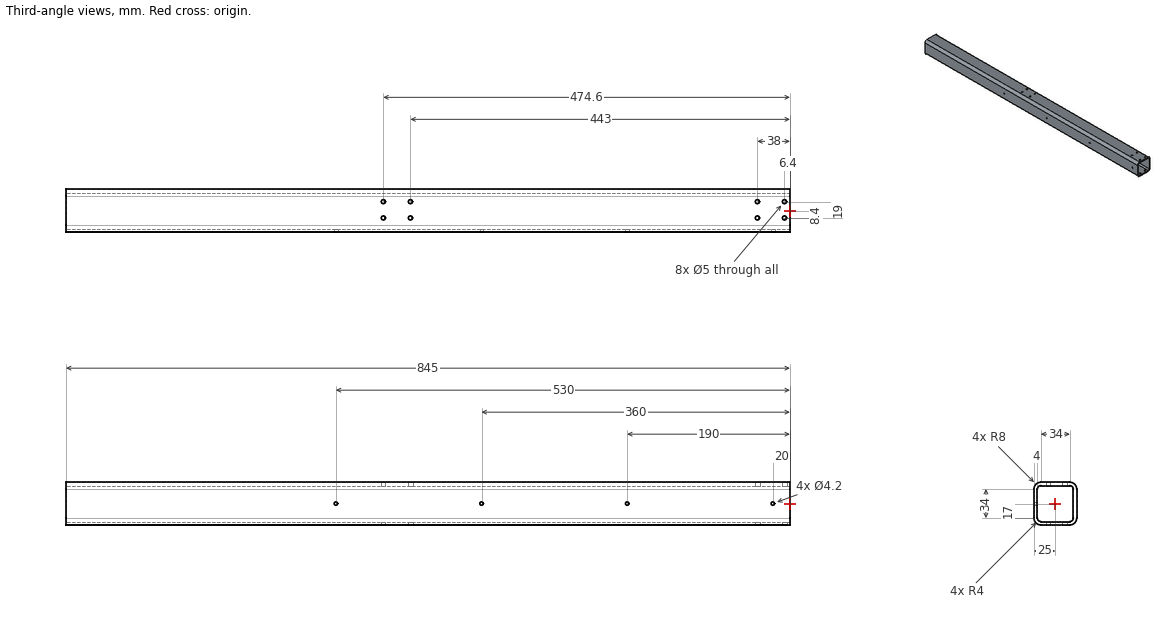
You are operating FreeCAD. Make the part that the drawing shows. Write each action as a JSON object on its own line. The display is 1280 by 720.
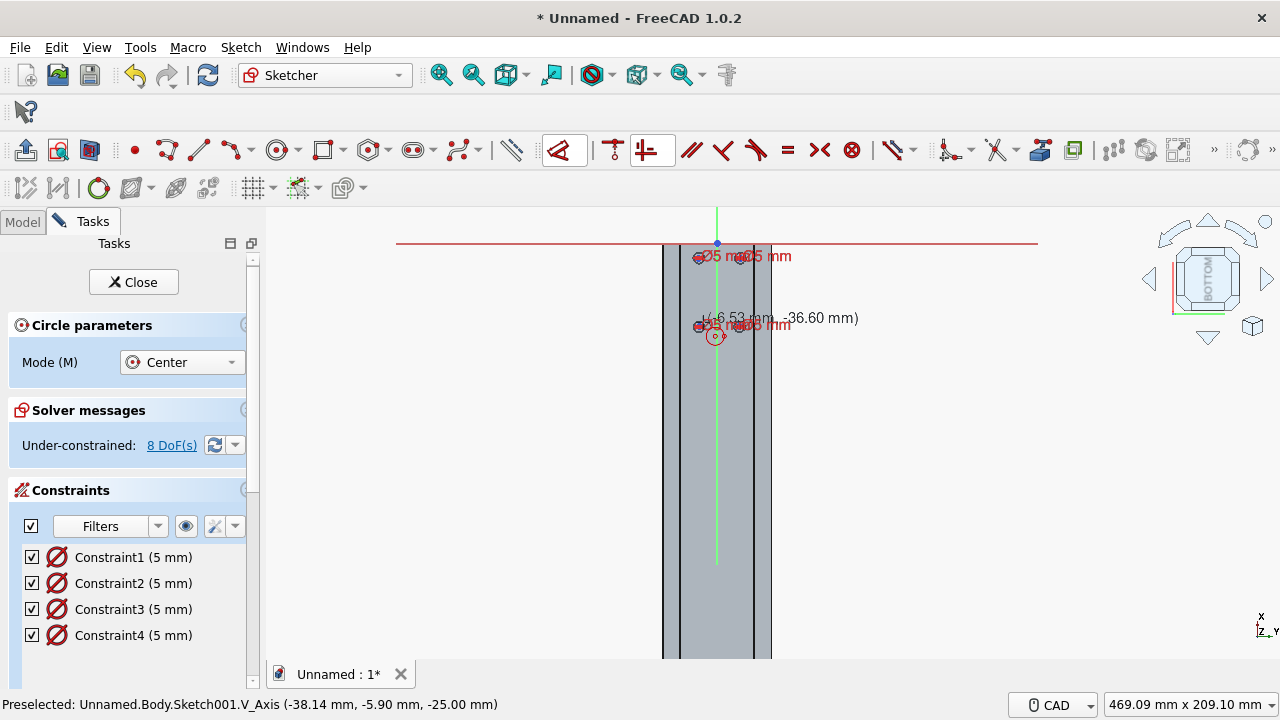
{"action": "scroll", "coordinate": [700, 326], "scroll_direction": "down", "scroll_amount": 7}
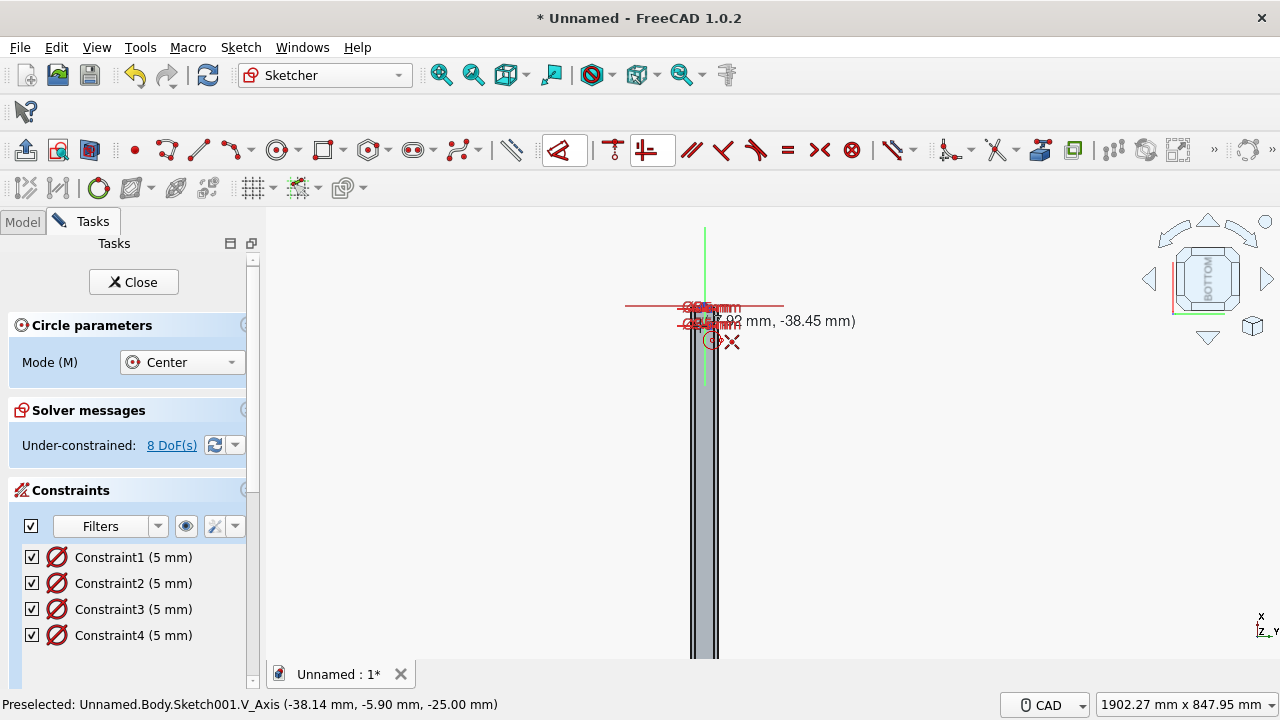
{"action": "scroll", "coordinate": [710, 542], "scroll_direction": "up", "scroll_amount": 15}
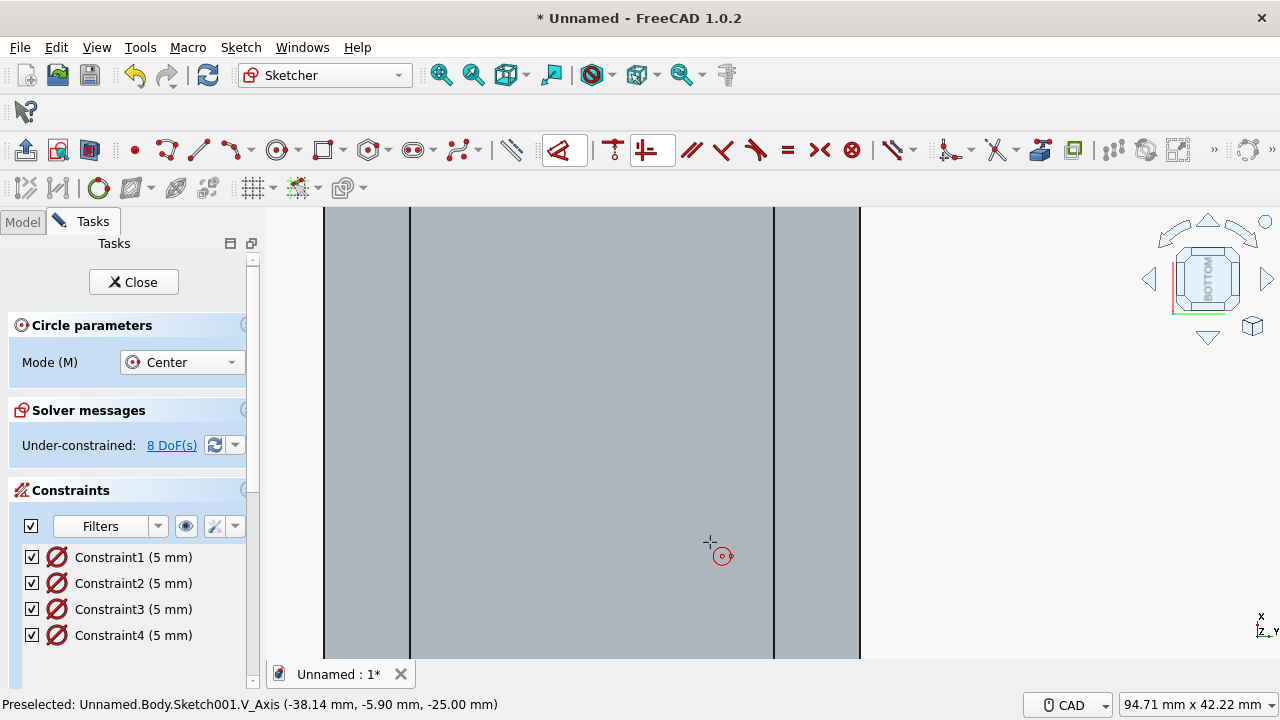
{"action": "scroll", "coordinate": [710, 543], "scroll_direction": "down", "scroll_amount": 15}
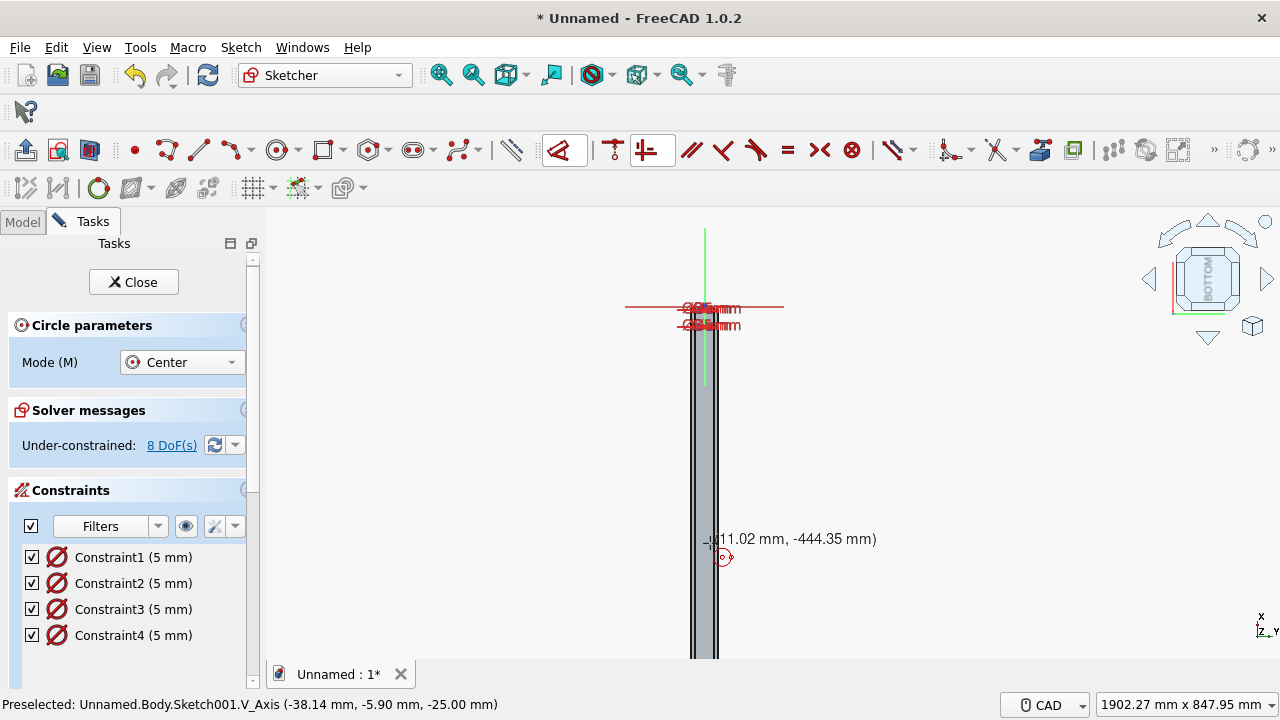
{"action": "scroll", "coordinate": [710, 543], "scroll_direction": "up", "scroll_amount": 6}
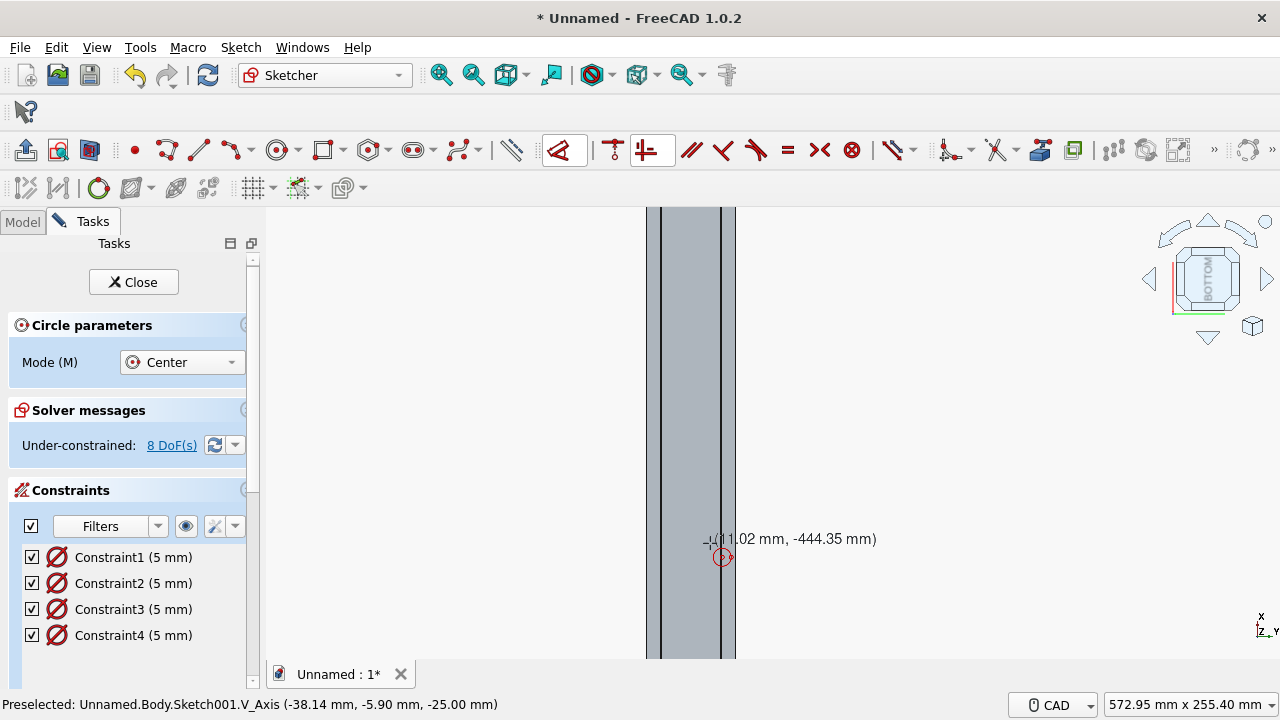
{"action": "left_click", "coordinate": [710, 541]}
{"action": "mouse_move", "coordinate": [713, 538]}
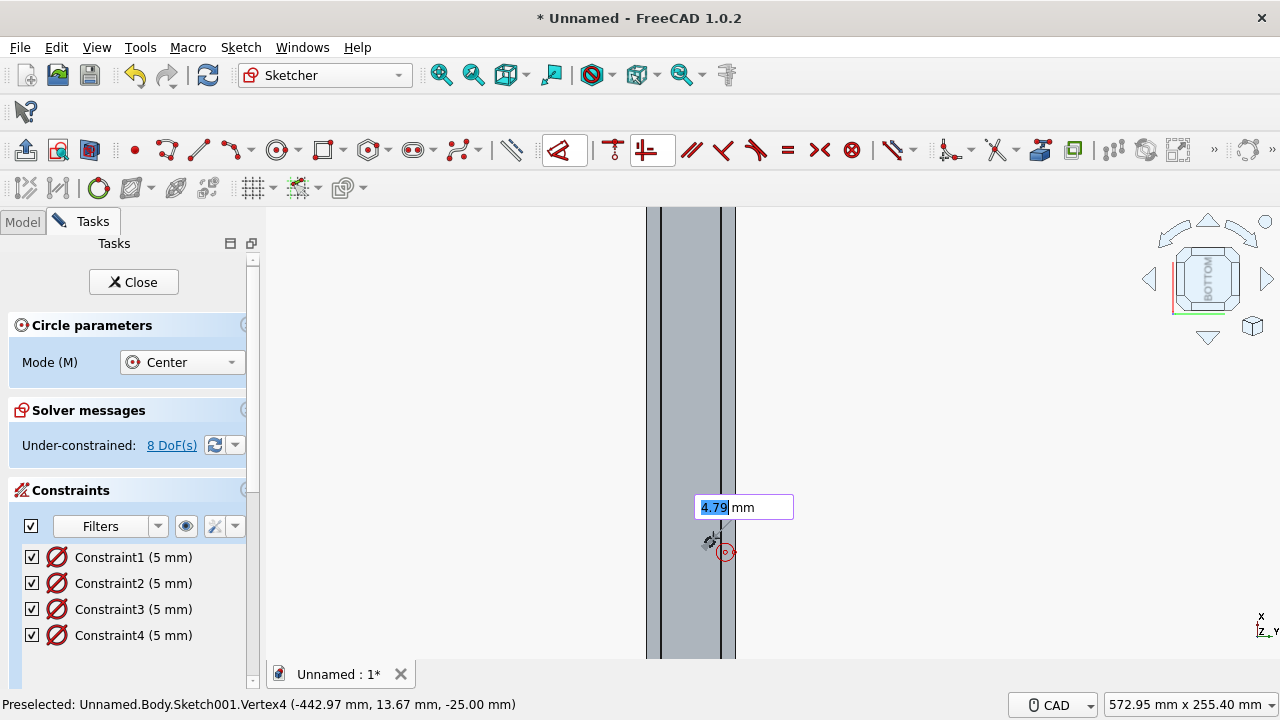
{"action": "type", "text": "5"}
{"action": "key", "text": "Return"}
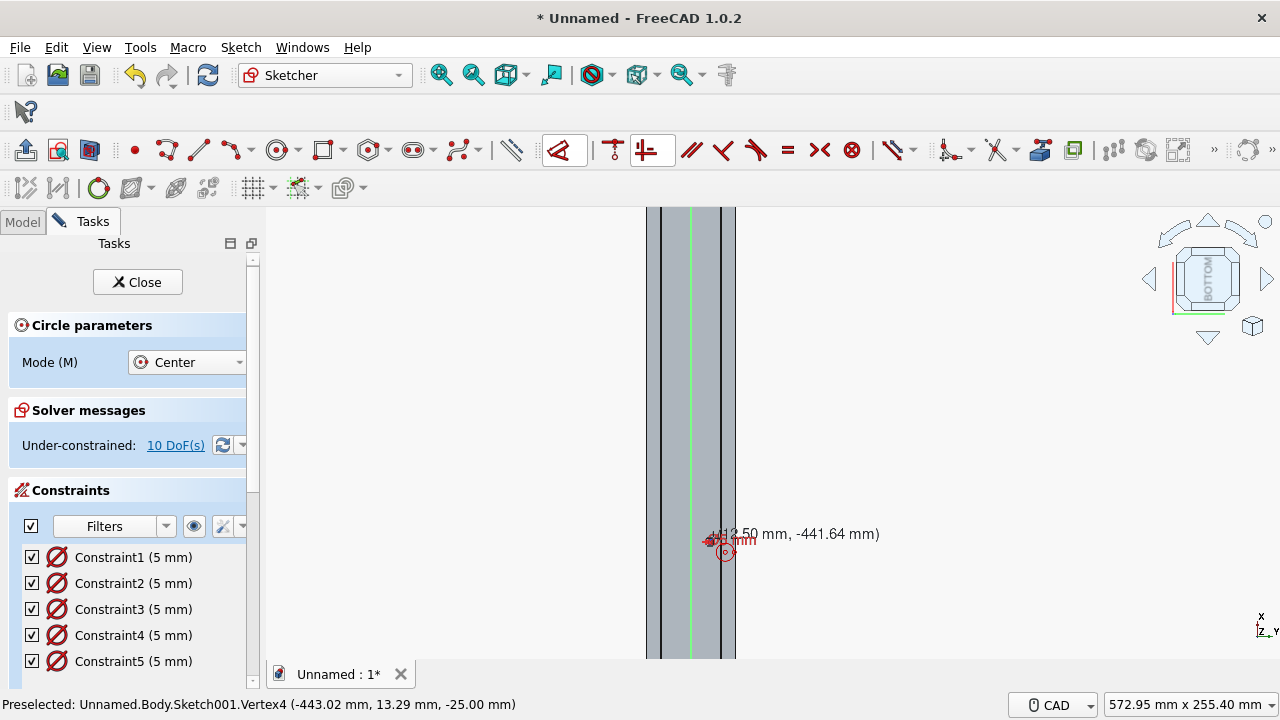
{"action": "scroll", "coordinate": [676, 541], "scroll_direction": "up", "scroll_amount": 9}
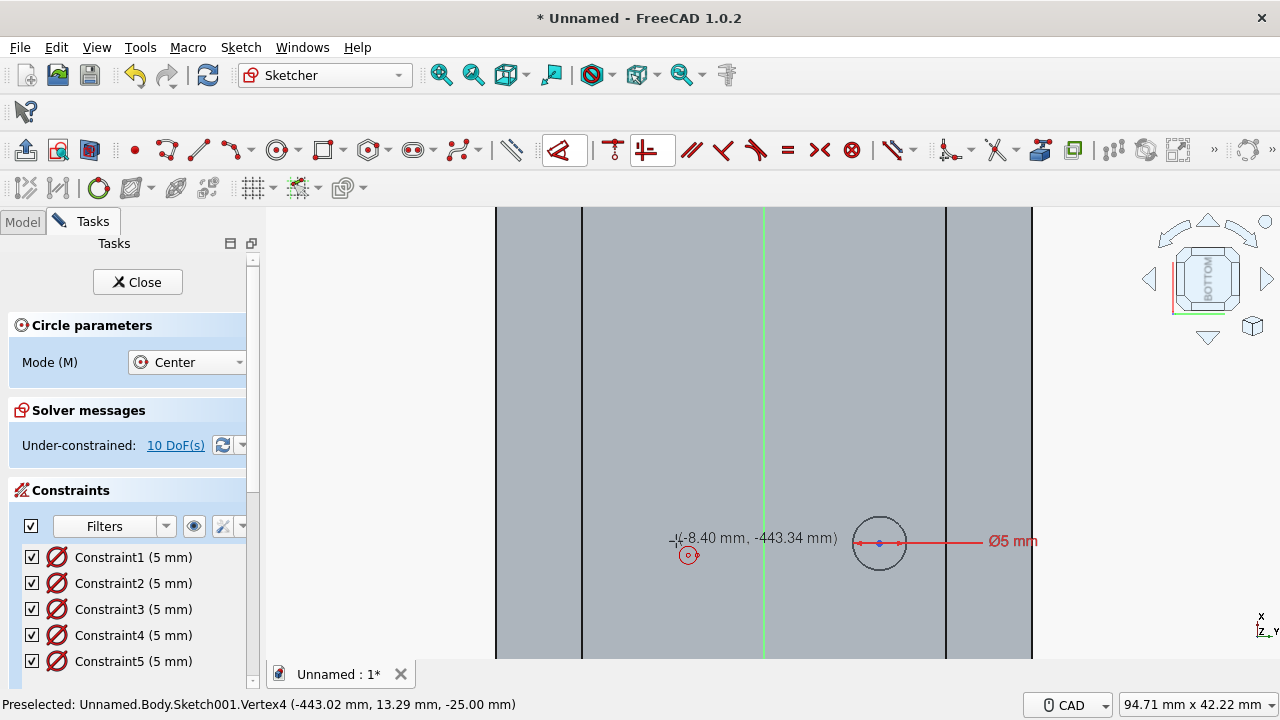
{"action": "scroll", "coordinate": [701, 542], "scroll_direction": "down", "scroll_amount": 15}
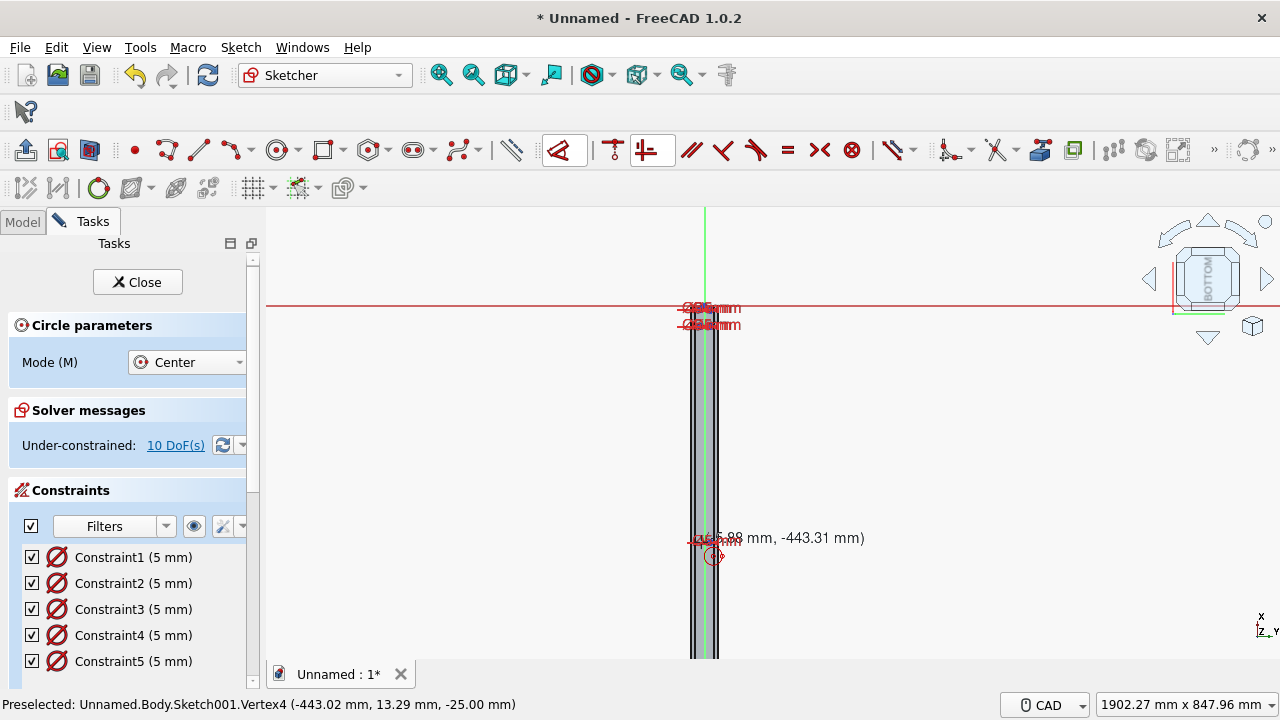
{"action": "scroll", "coordinate": [700, 543], "scroll_direction": "up", "scroll_amount": 7}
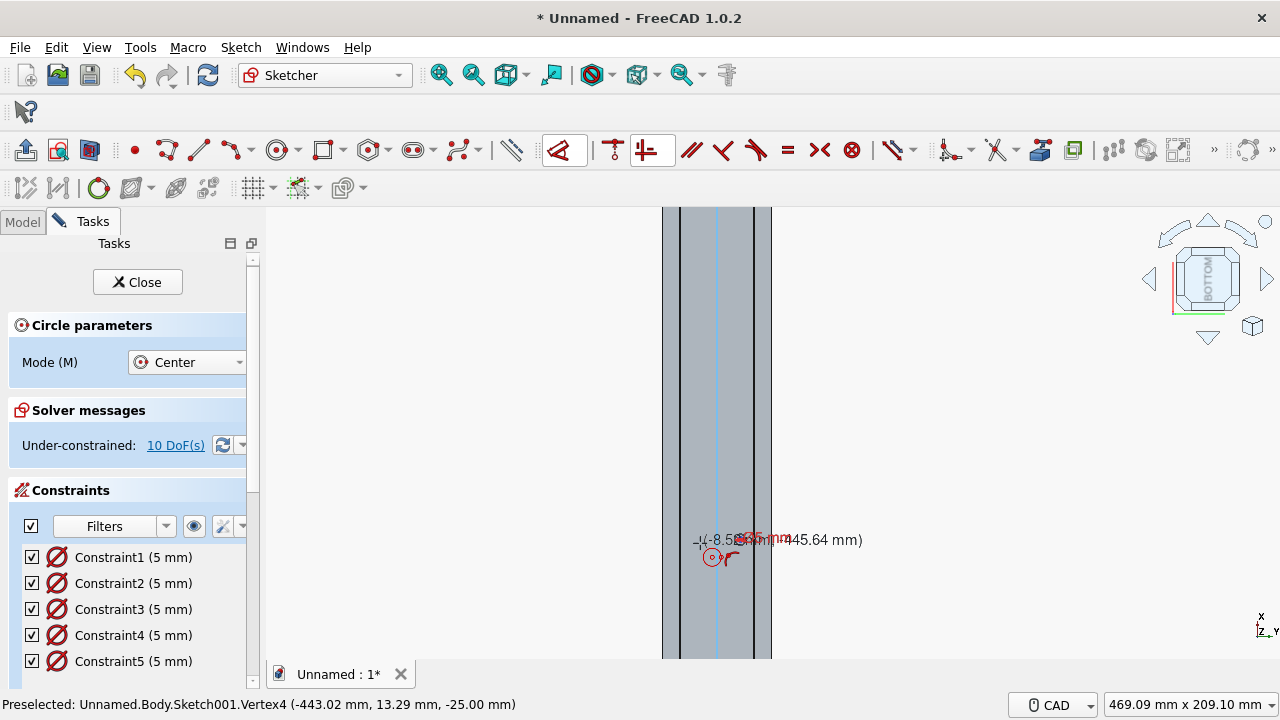
{"action": "left_click", "coordinate": [699, 539]}
{"action": "mouse_move", "coordinate": [703, 535]}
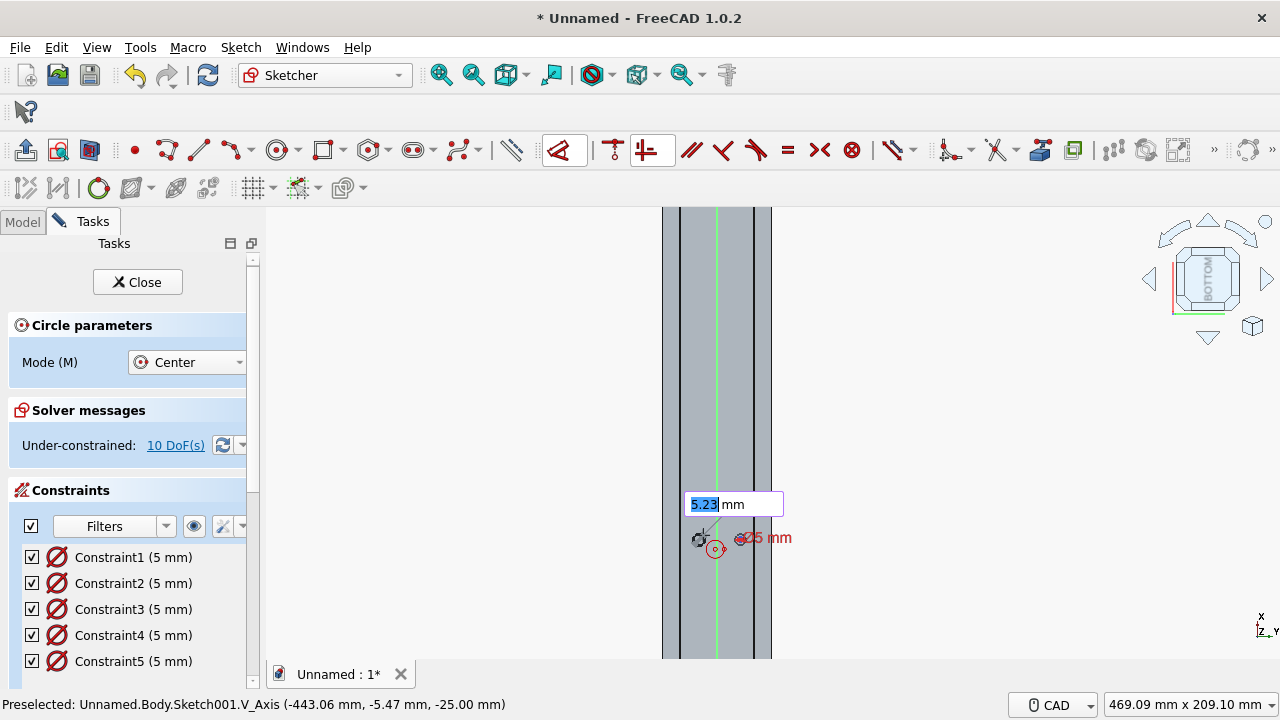
{"action": "type", "text": "5"}
{"action": "key", "text": "Return"}